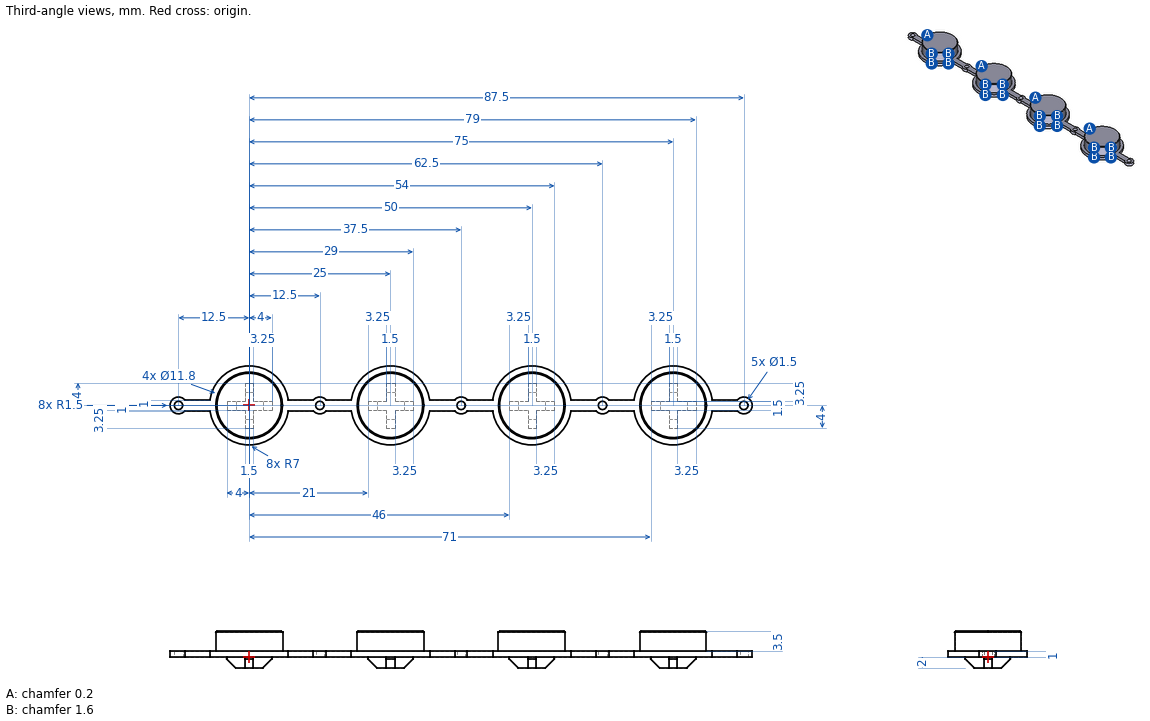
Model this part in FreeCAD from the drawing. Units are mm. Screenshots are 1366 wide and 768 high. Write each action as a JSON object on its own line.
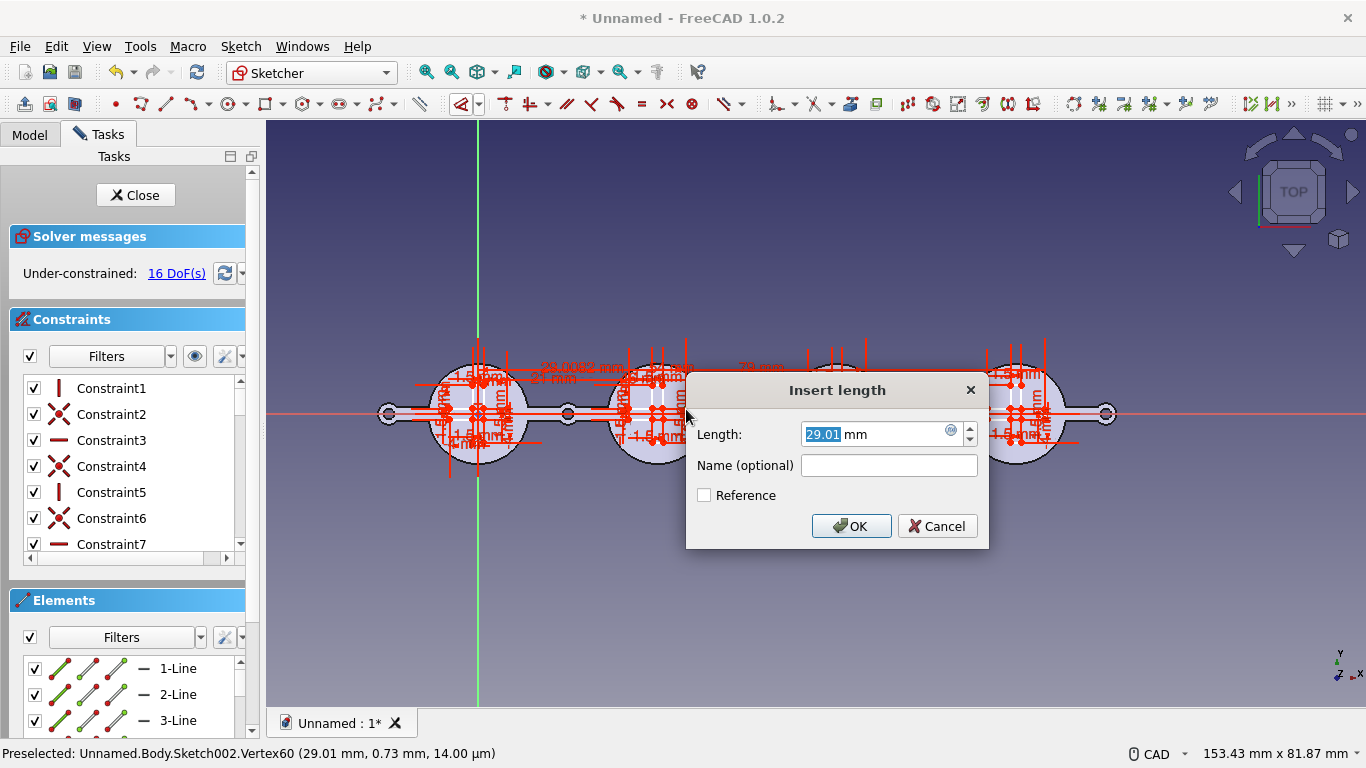
{"action": "type", "text": "29"}
{"action": "key", "text": "Return"}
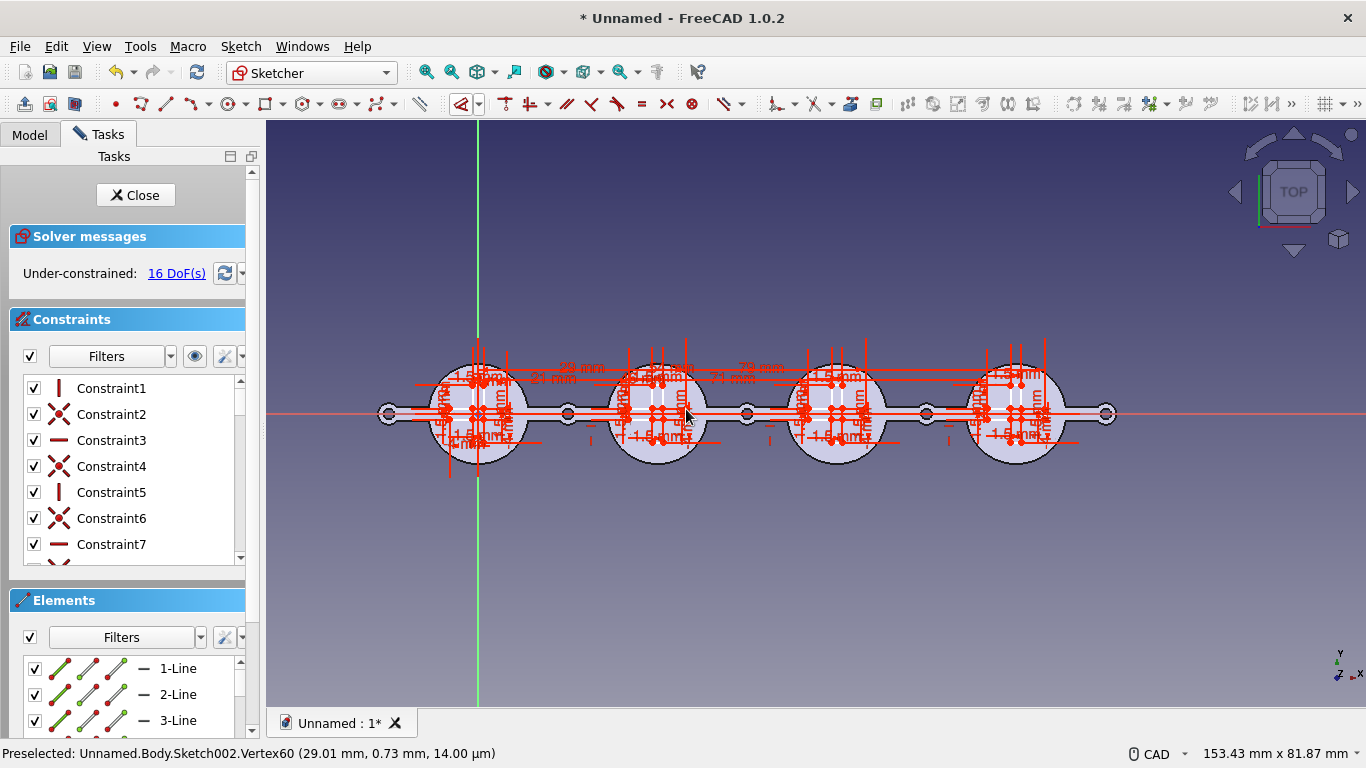
{"action": "scroll", "coordinate": [994, 409], "scroll_direction": "up", "scroll_amount": 5}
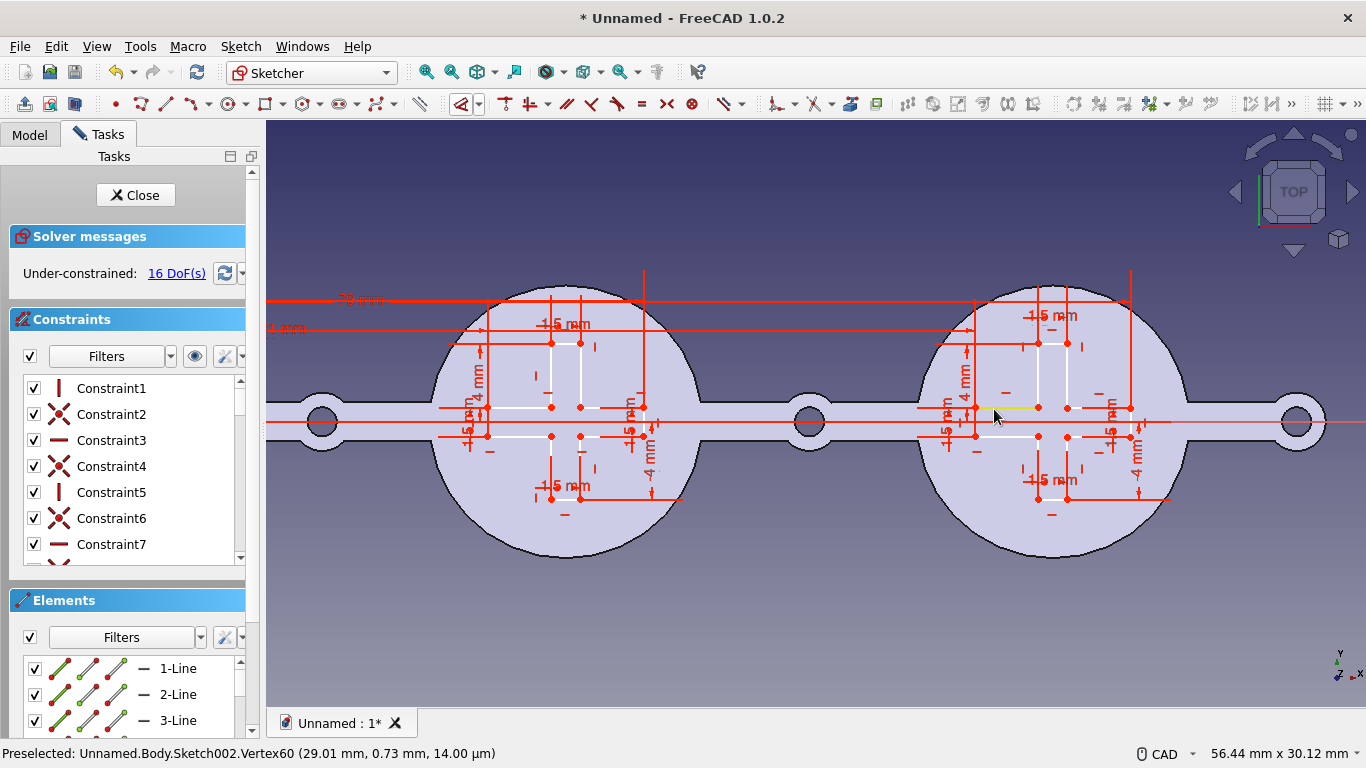
{"action": "left_click", "coordinate": [994, 408]}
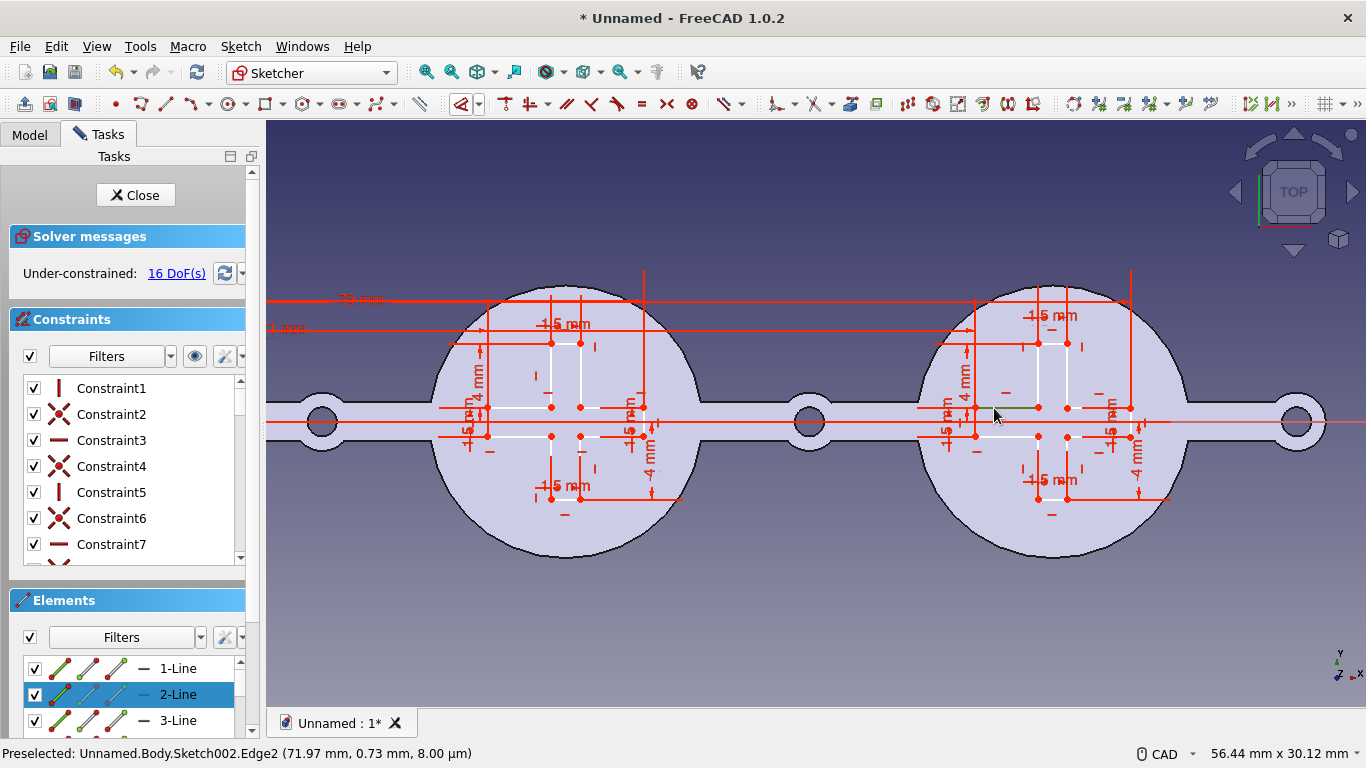
{"action": "left_click", "coordinate": [478, 104]}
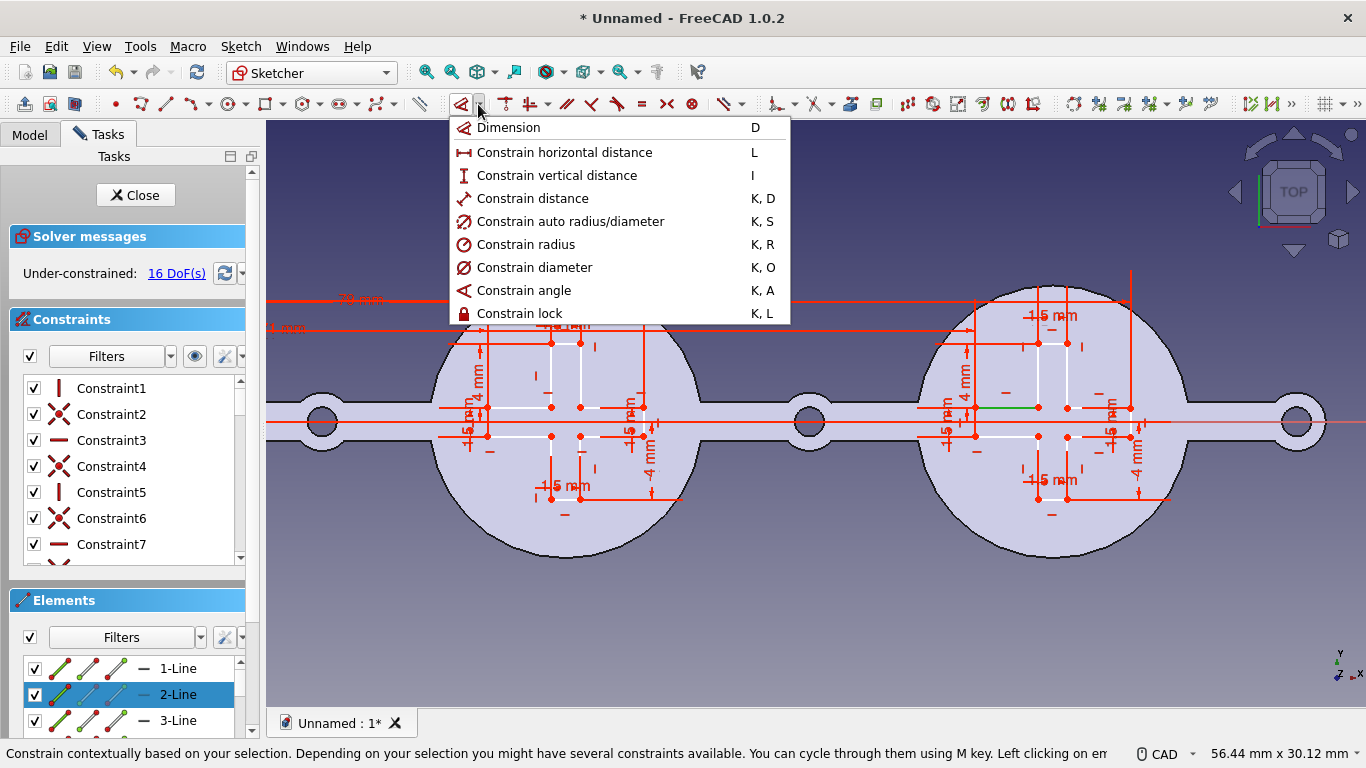
{"action": "left_click", "coordinate": [620, 152]}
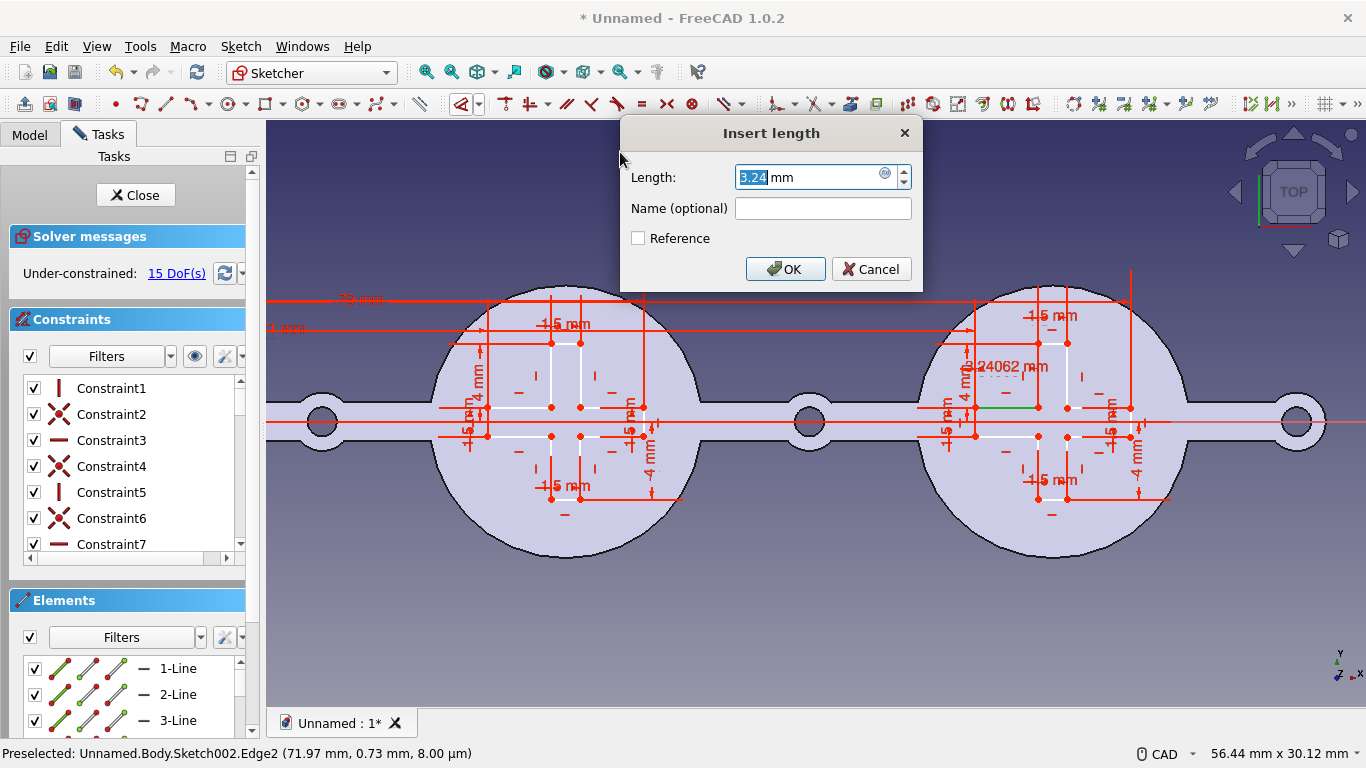
{"action": "type", "text": "3.25"}
{"action": "key", "text": "Return"}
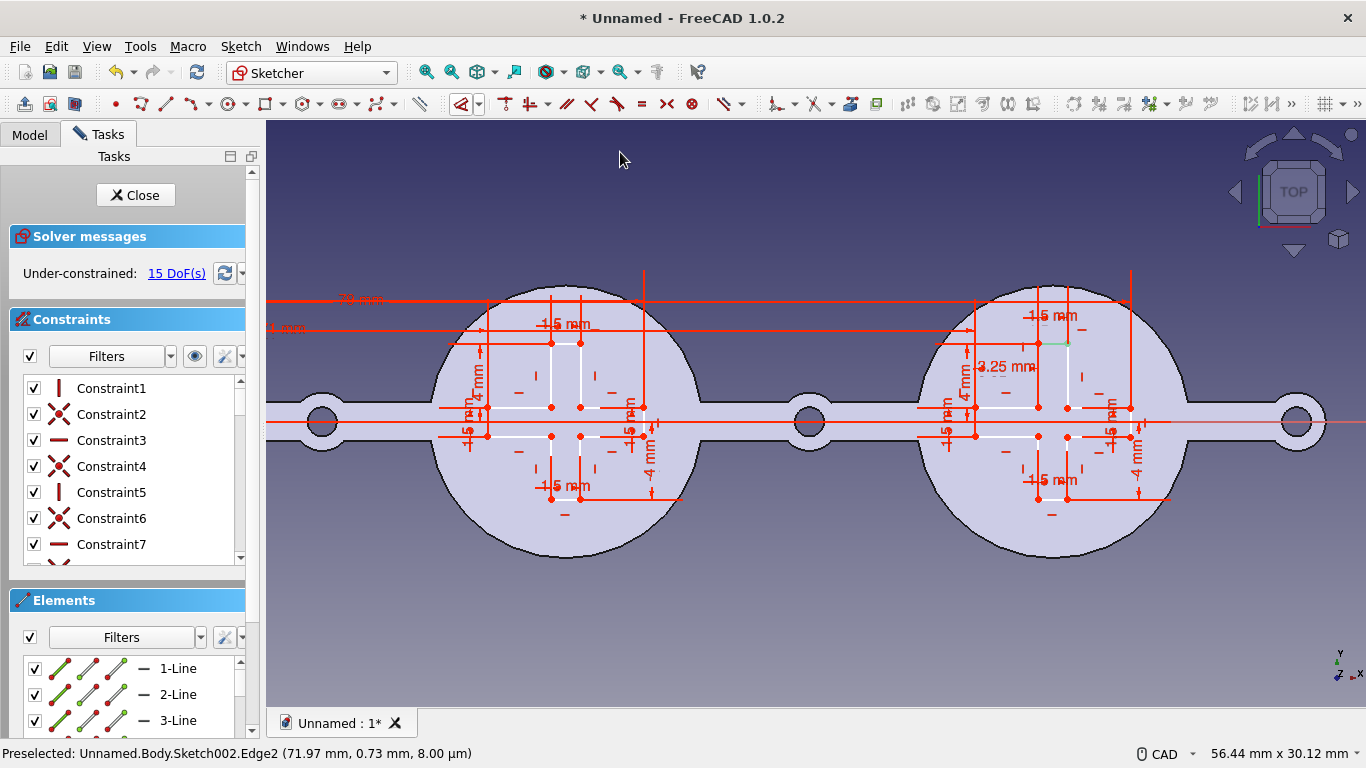
{"action": "left_click", "coordinate": [1038, 389]}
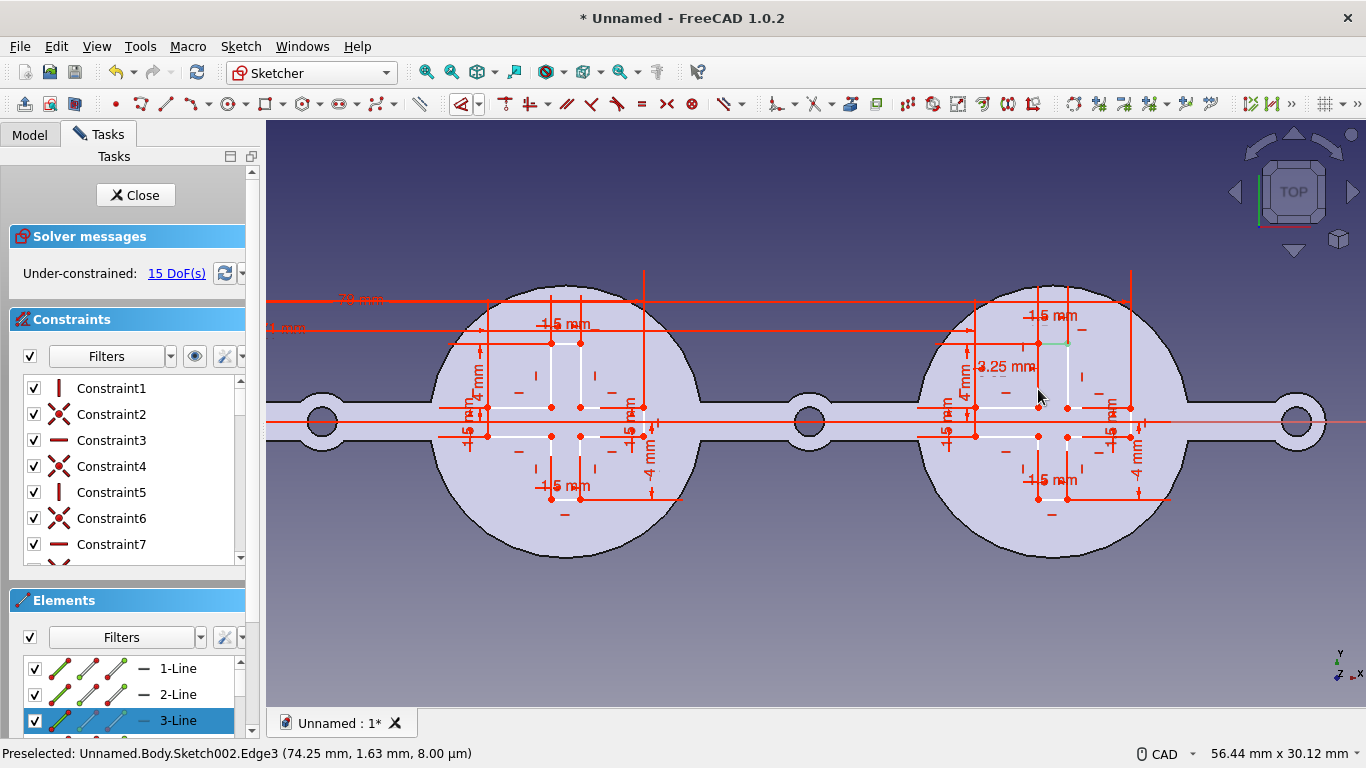
{"action": "key", "text": "i"}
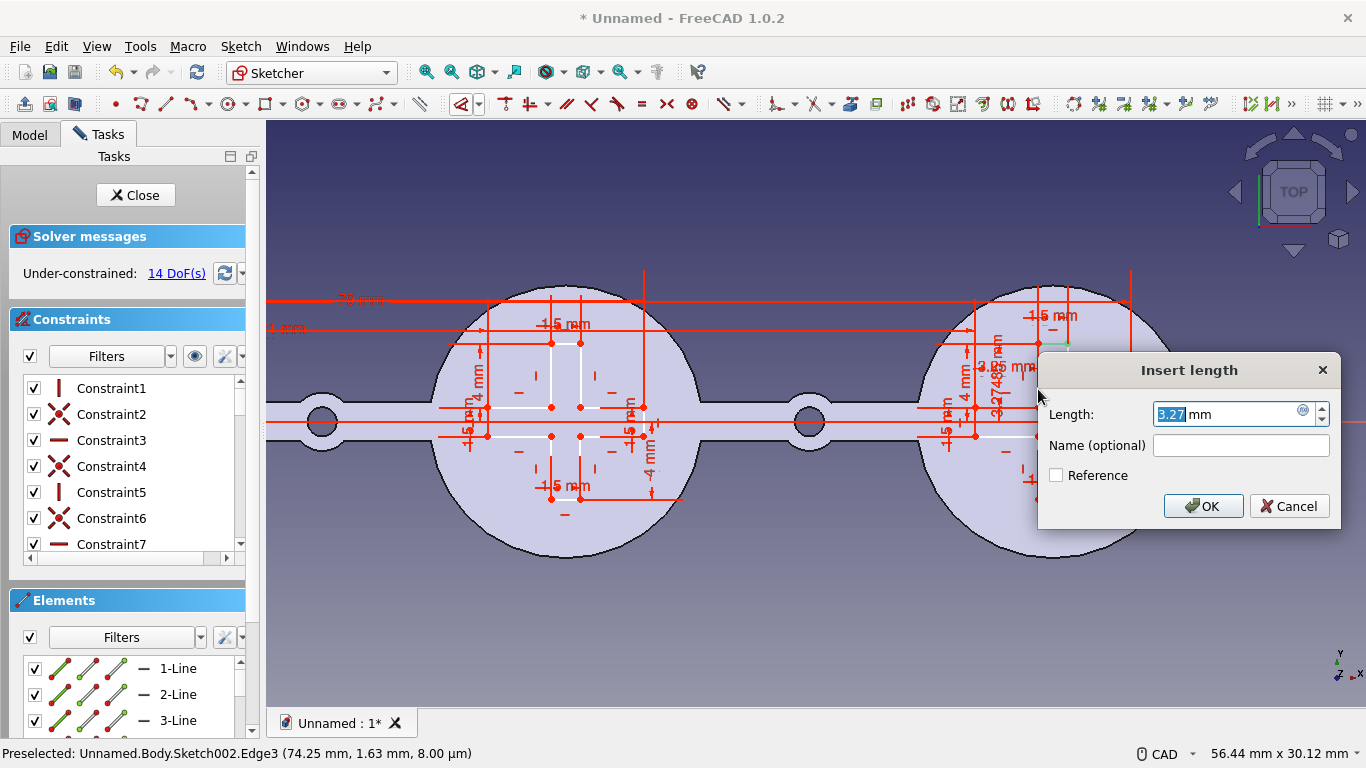
{"action": "type", "text": "3.25"}
{"action": "key", "text": "Return"}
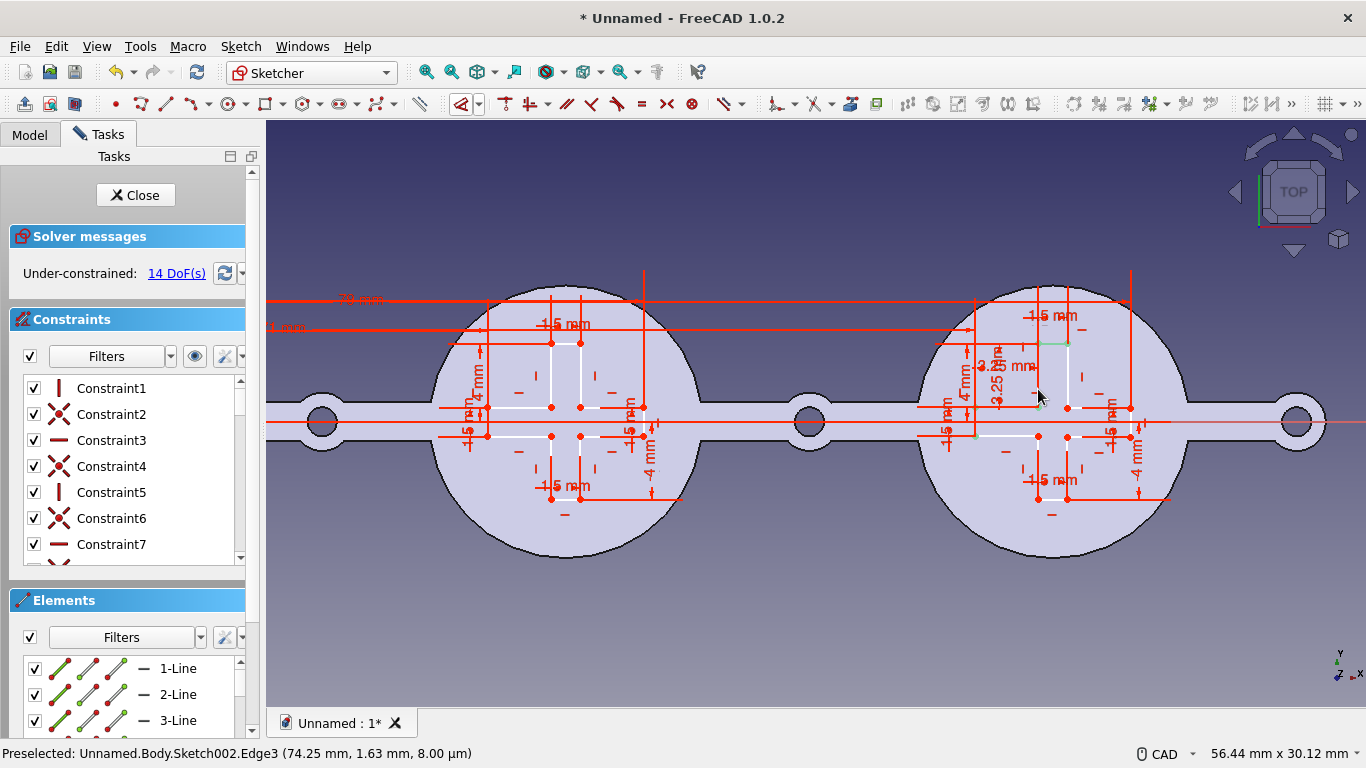
{"action": "left_click", "coordinate": [1068, 363]}